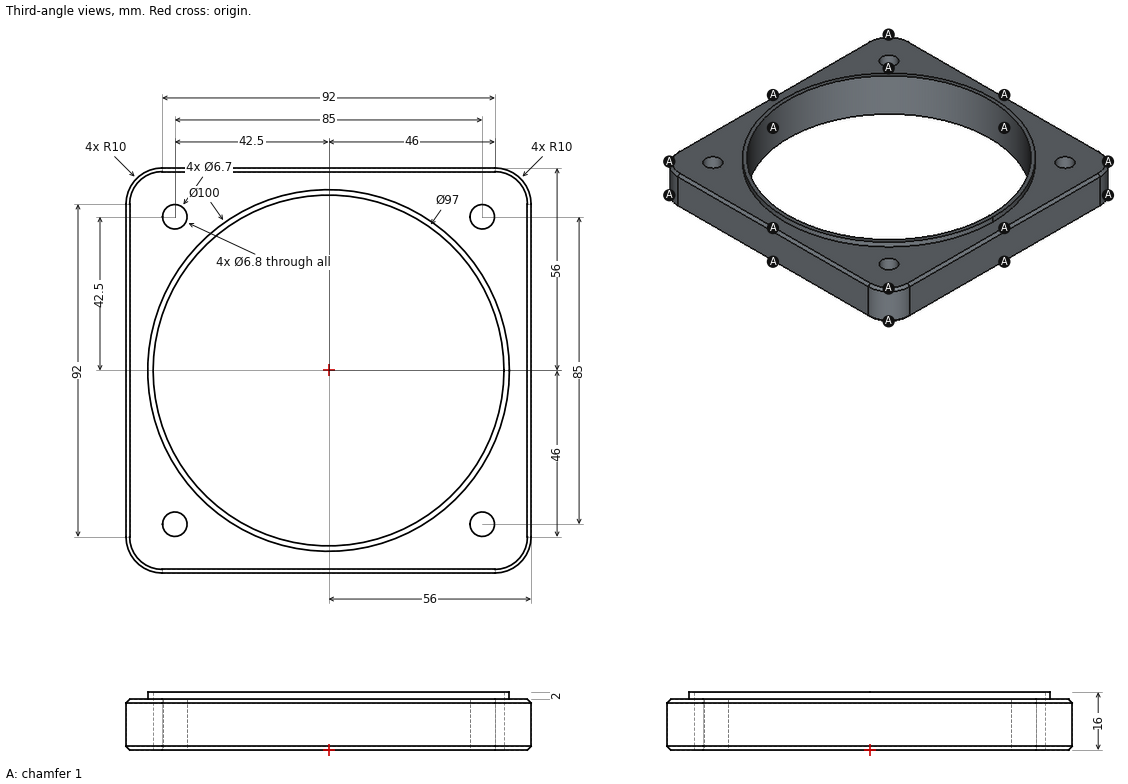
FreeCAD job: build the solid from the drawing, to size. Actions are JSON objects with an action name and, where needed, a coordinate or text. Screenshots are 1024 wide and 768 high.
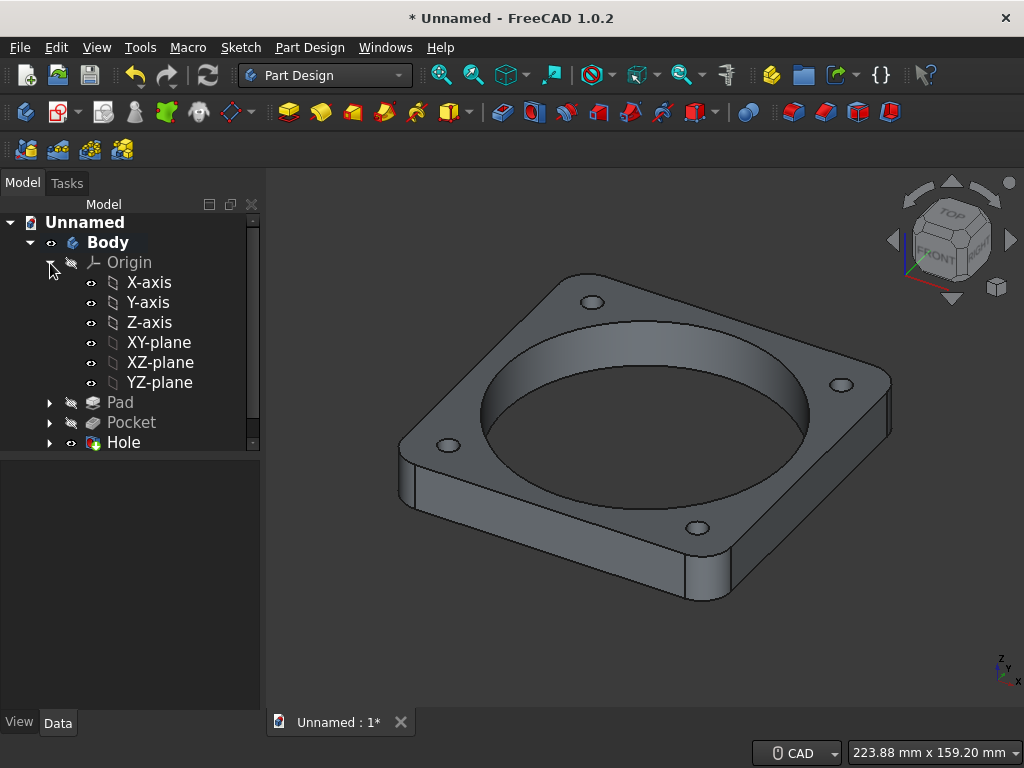
{"action": "left_click", "coordinate": [136, 343]}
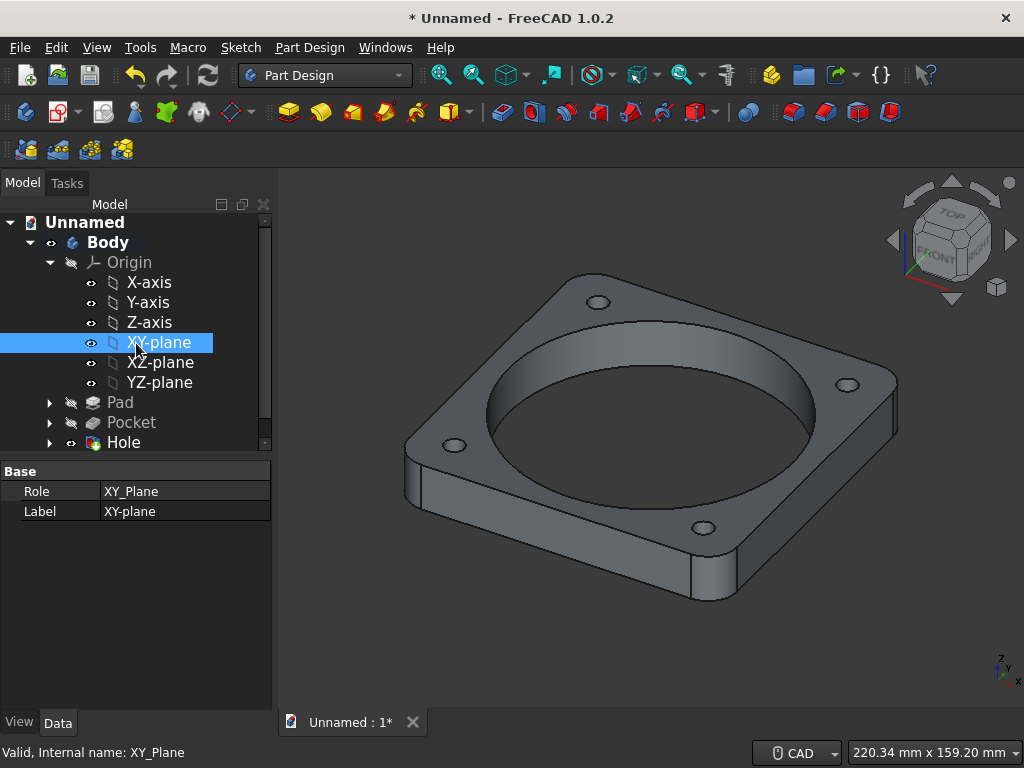
{"action": "left_click", "coordinate": [232, 112]}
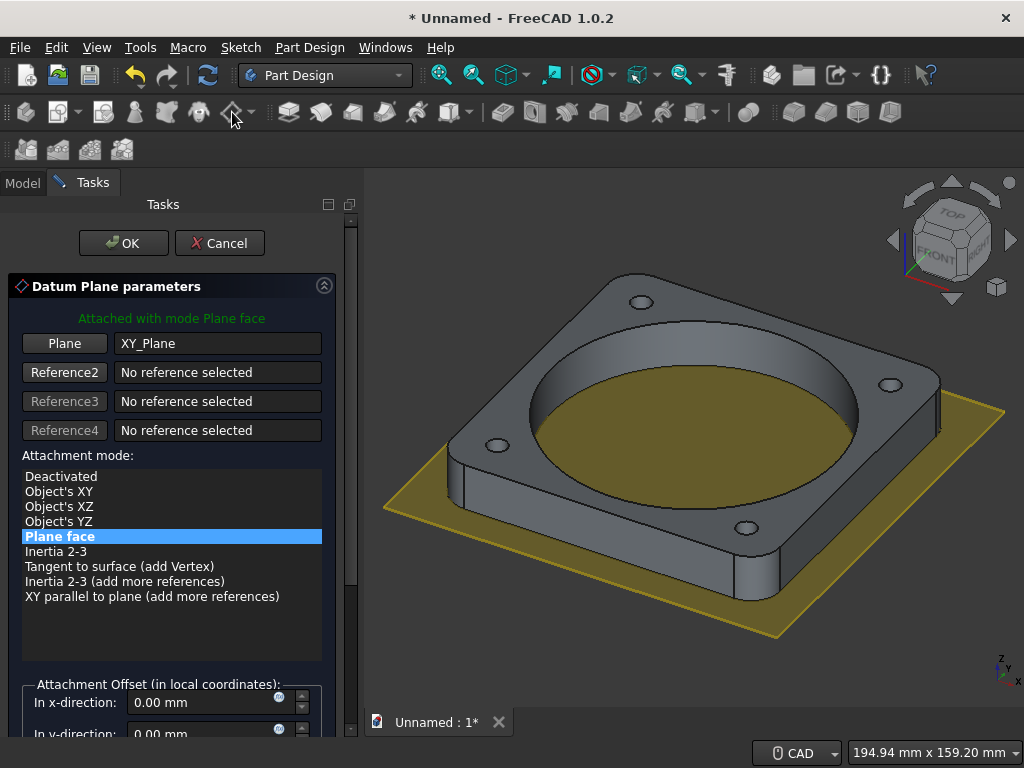
{"action": "scroll", "coordinate": [351, 475], "scroll_direction": "down", "scroll_amount": 2}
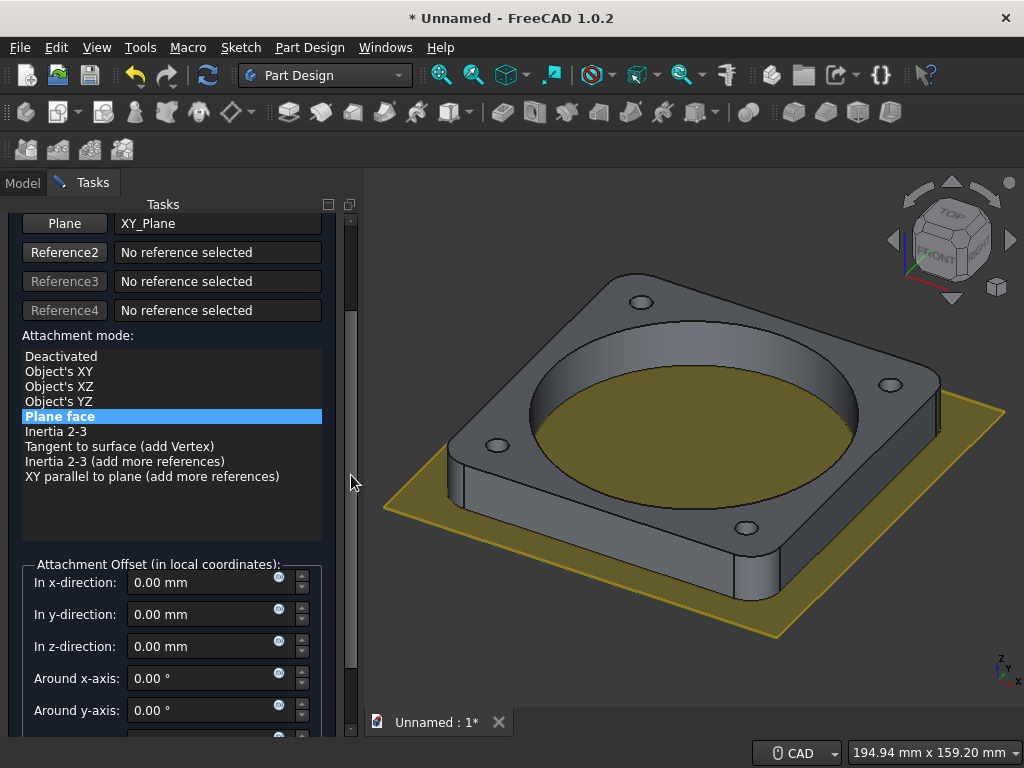
{"action": "triple_click", "coordinate": [210, 646]}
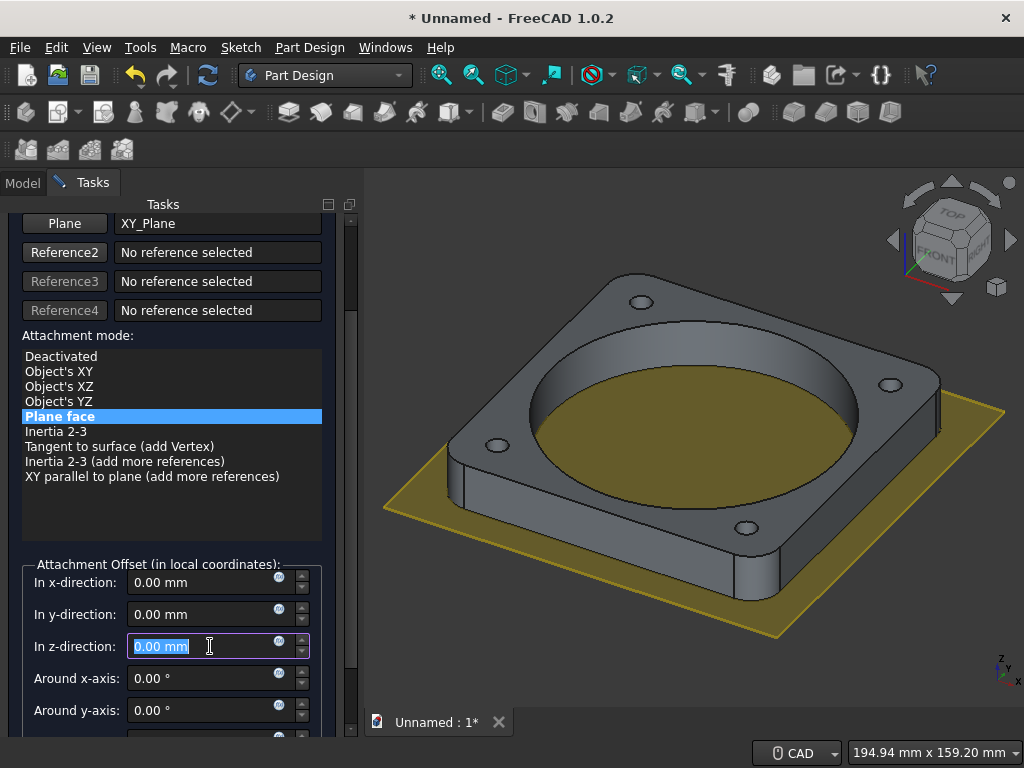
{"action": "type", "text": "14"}
{"action": "key", "text": "Tab"}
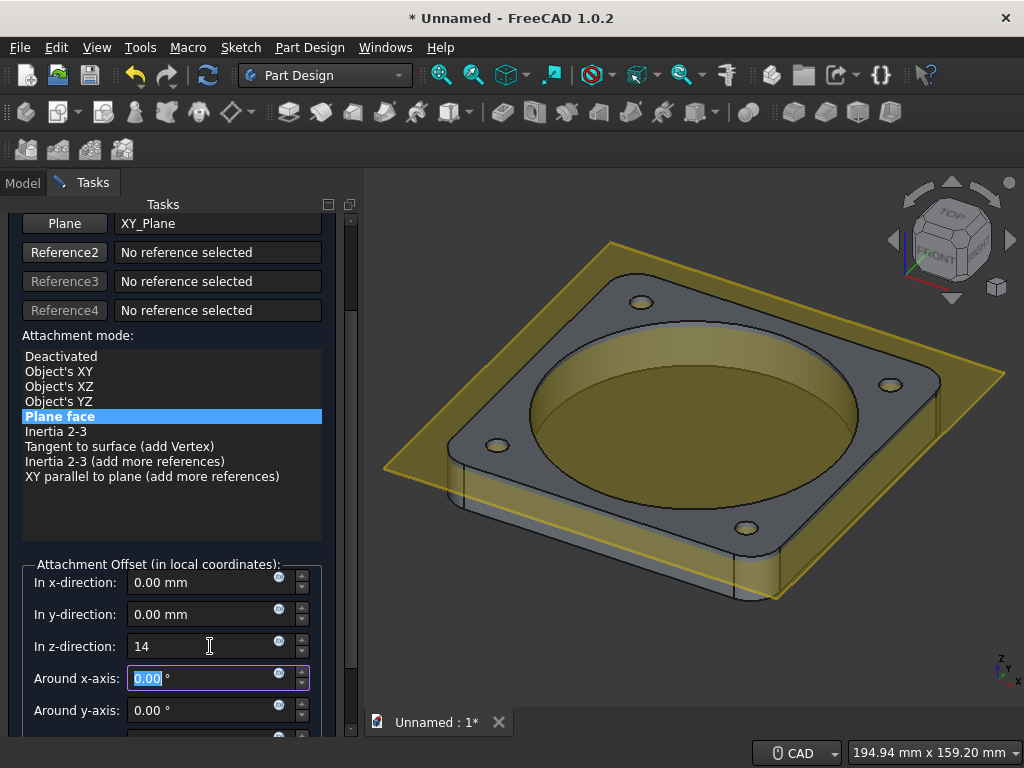
{"action": "scroll", "coordinate": [351, 475], "scroll_direction": "up", "scroll_amount": 3}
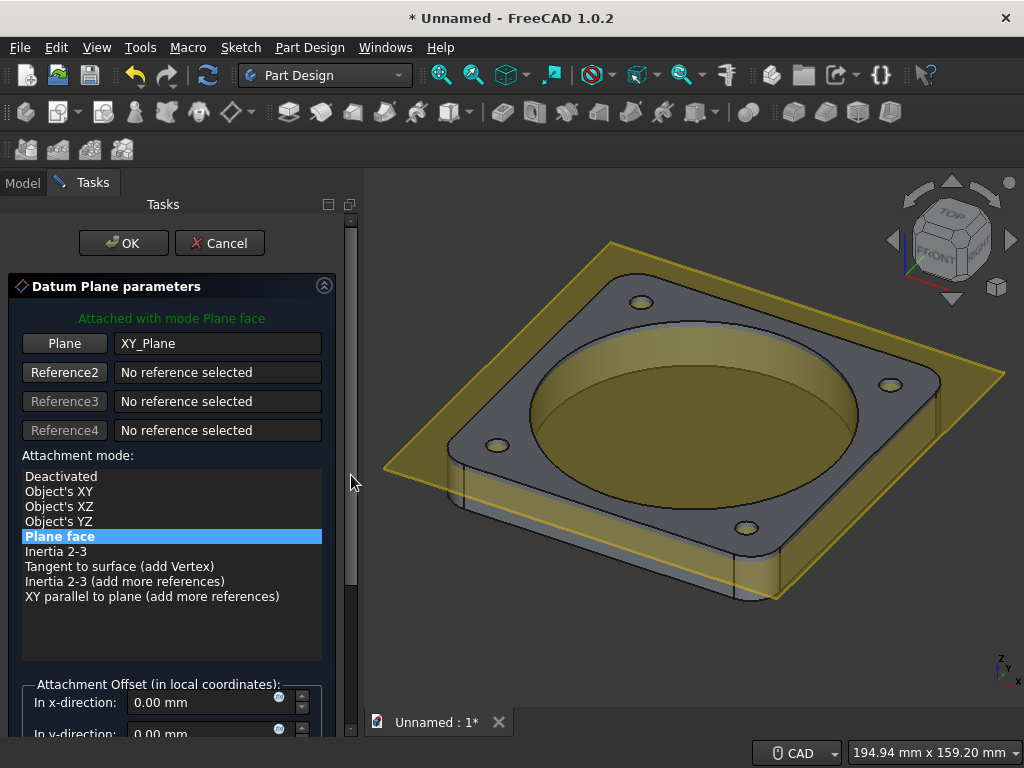
{"action": "left_click", "coordinate": [124, 243]}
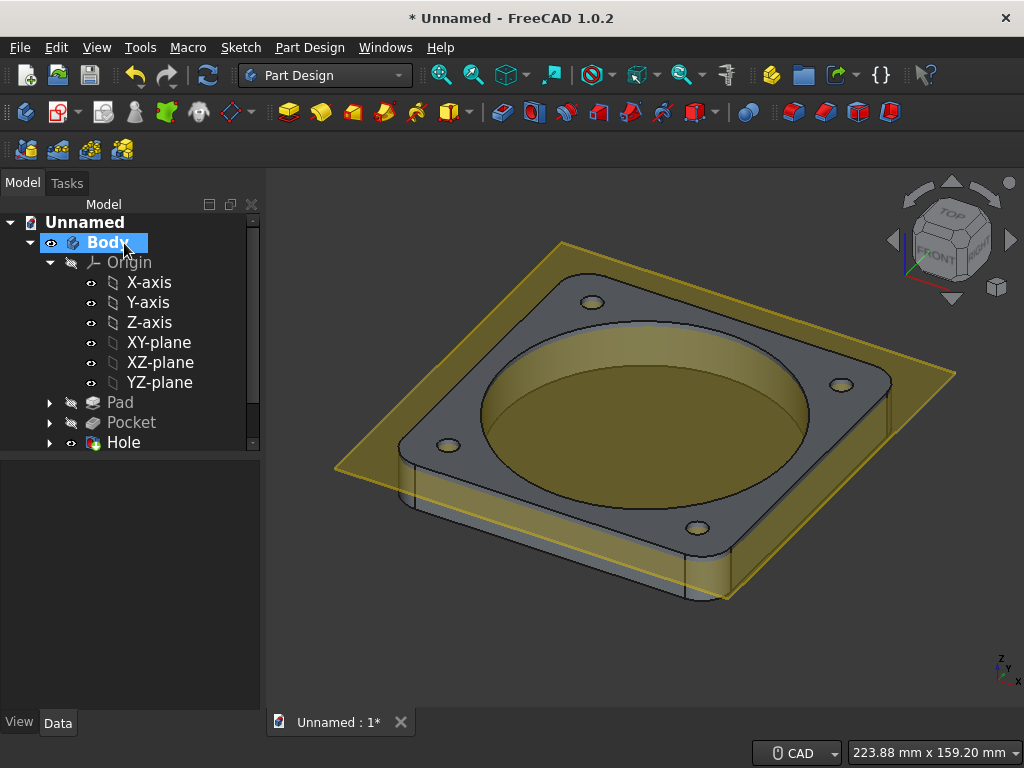
{"action": "scroll", "coordinate": [100, 338], "scroll_direction": "down", "scroll_amount": 3}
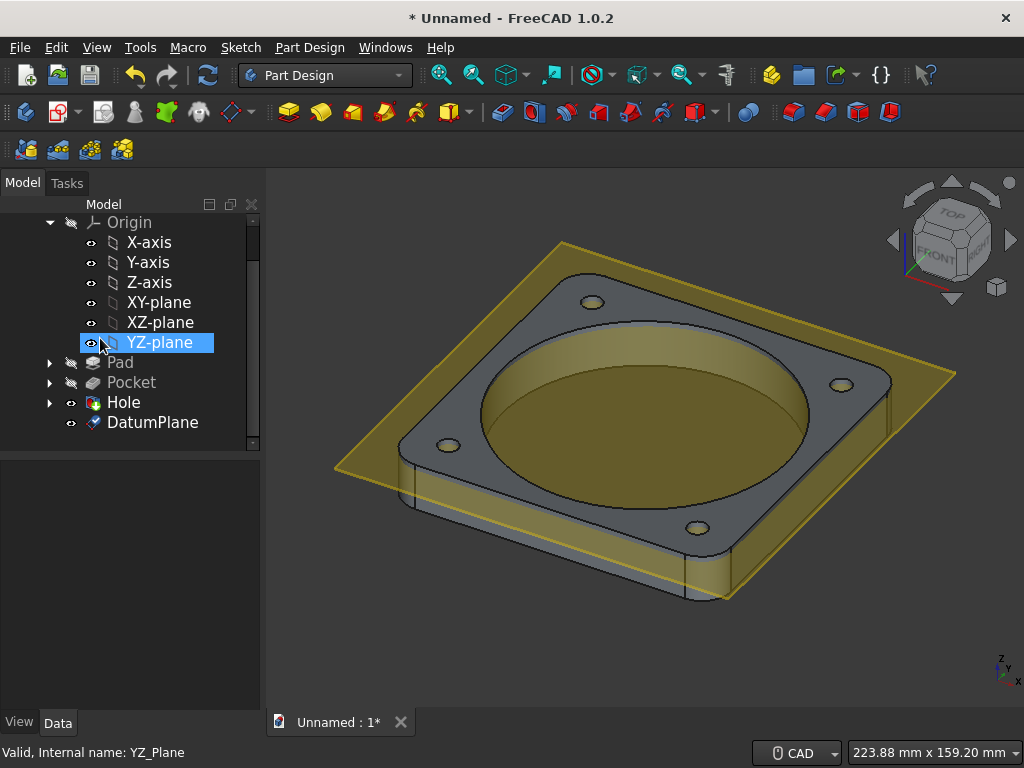
{"action": "left_click", "coordinate": [116, 423]}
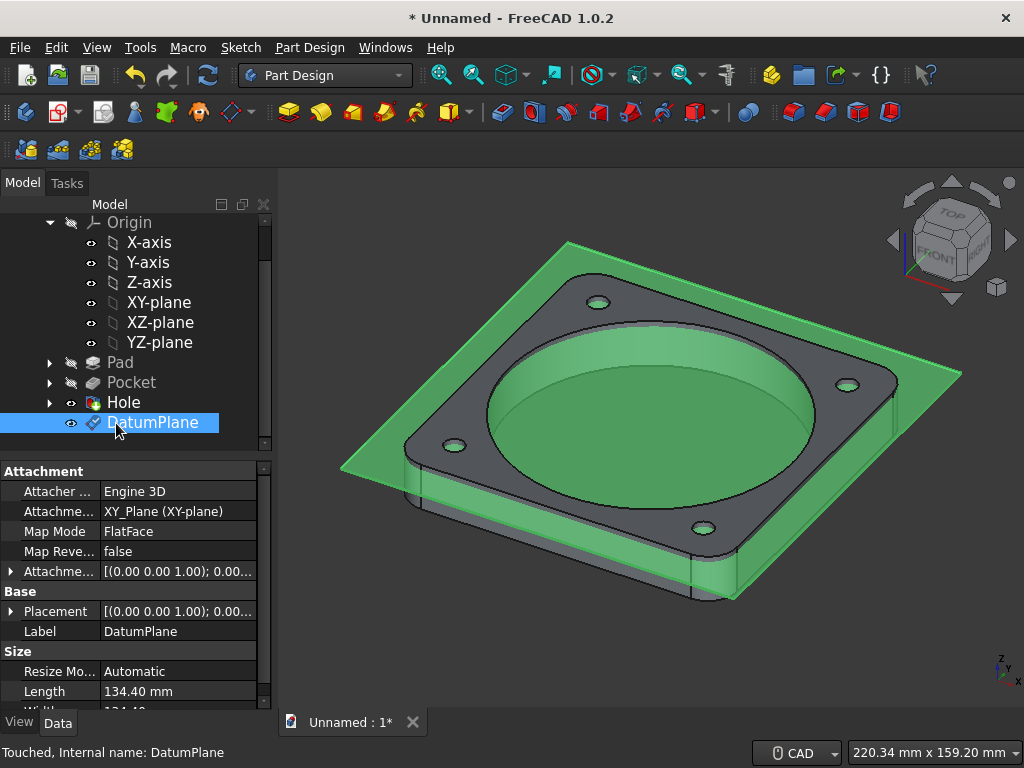
{"action": "left_click", "coordinate": [58, 112]}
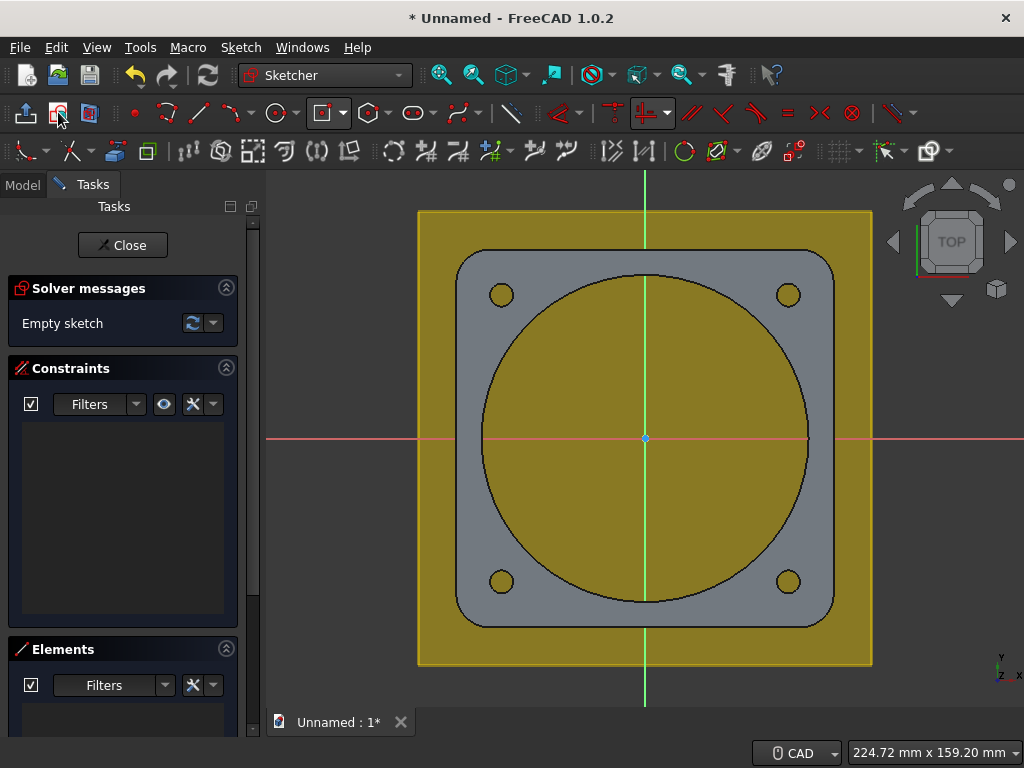
{"action": "left_click", "coordinate": [90, 114]}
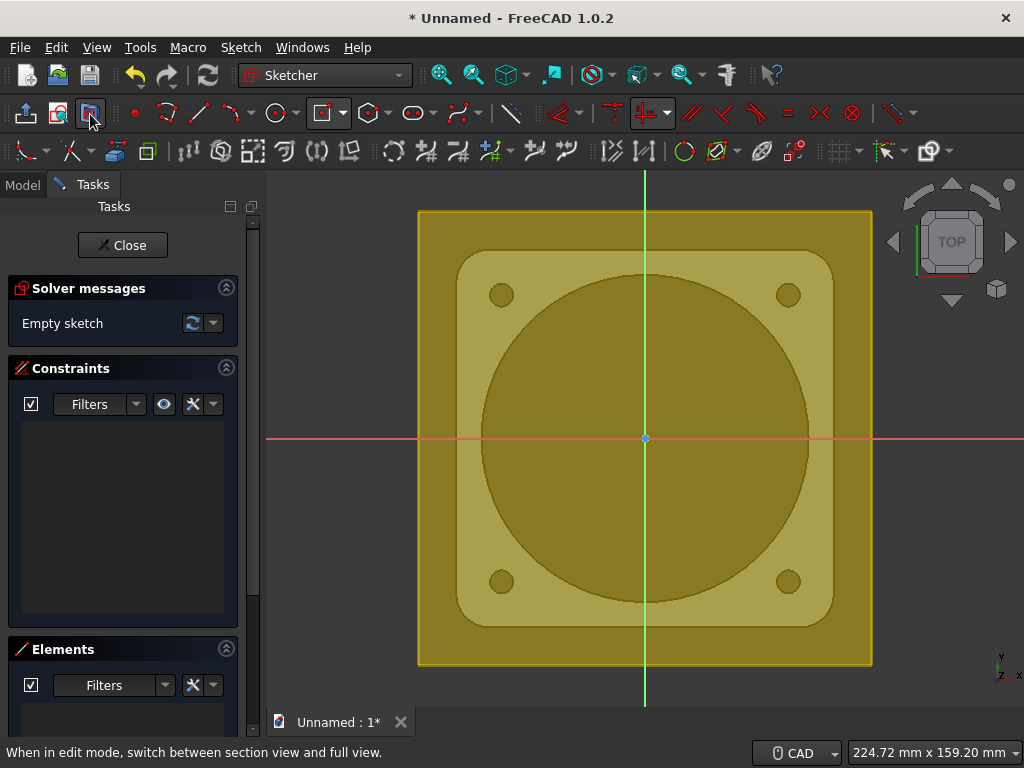
{"action": "left_click", "coordinate": [200, 114]}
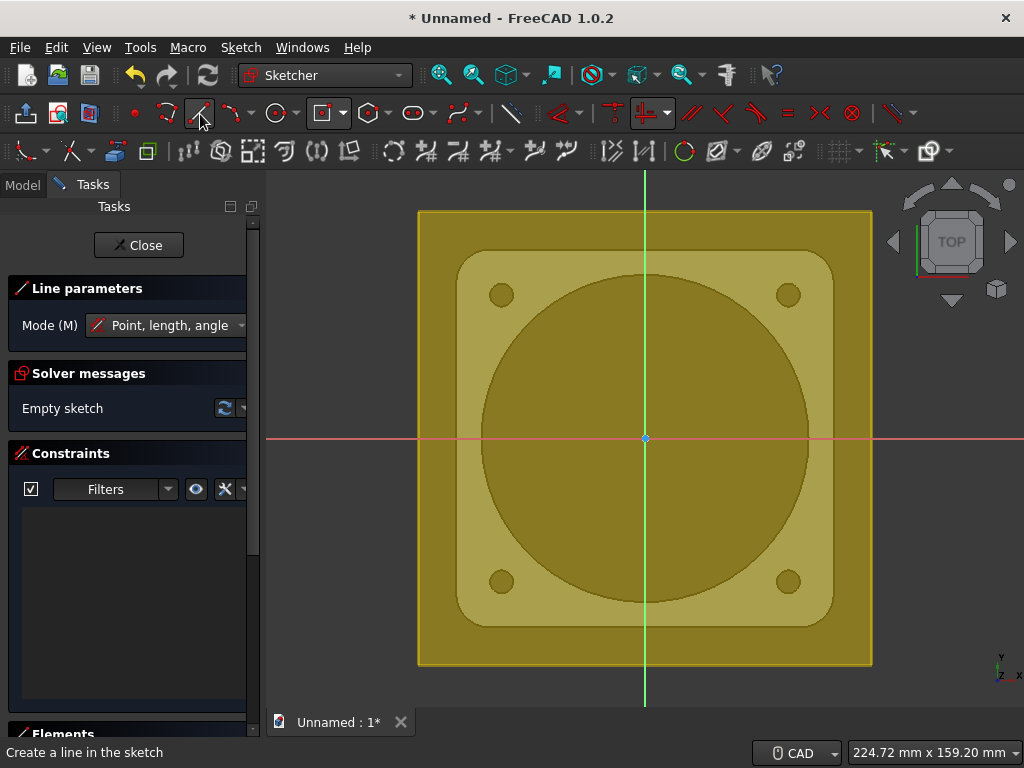
{"action": "left_click", "coordinate": [834, 594]}
{"action": "left_click", "coordinate": [834, 283]}